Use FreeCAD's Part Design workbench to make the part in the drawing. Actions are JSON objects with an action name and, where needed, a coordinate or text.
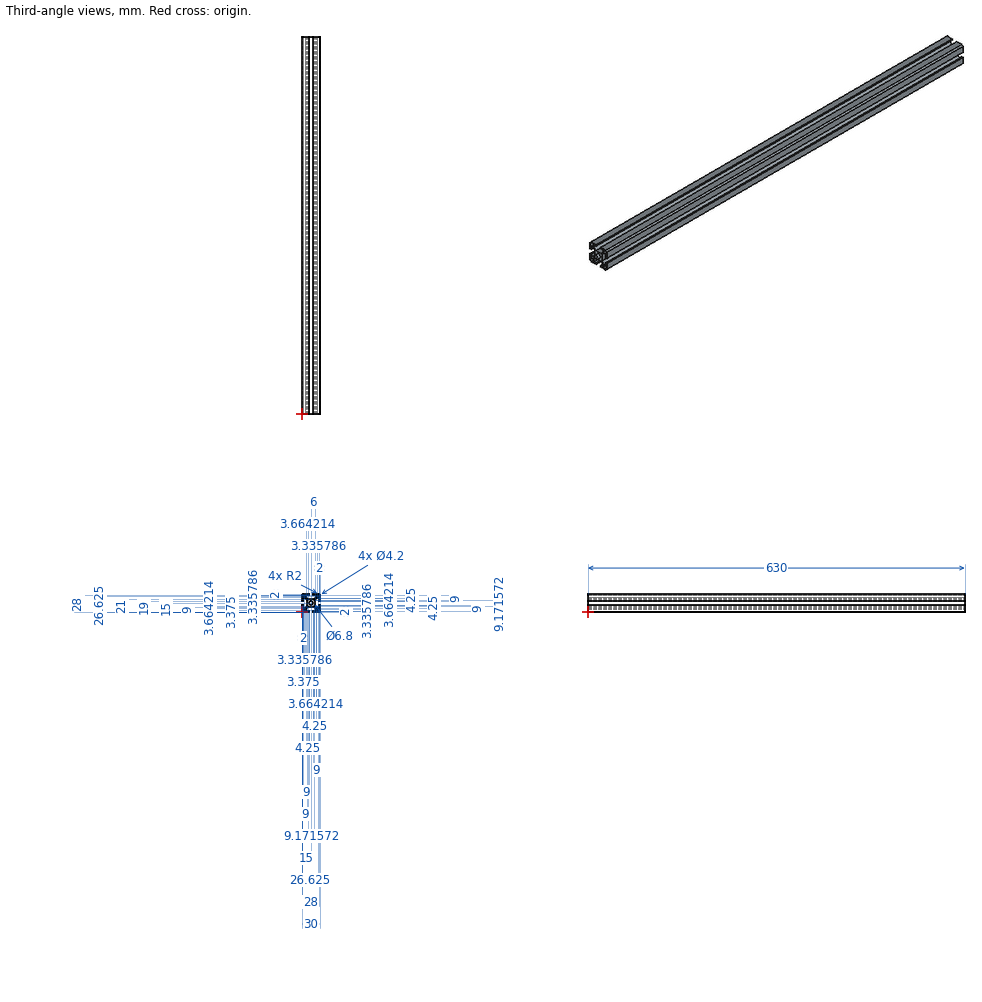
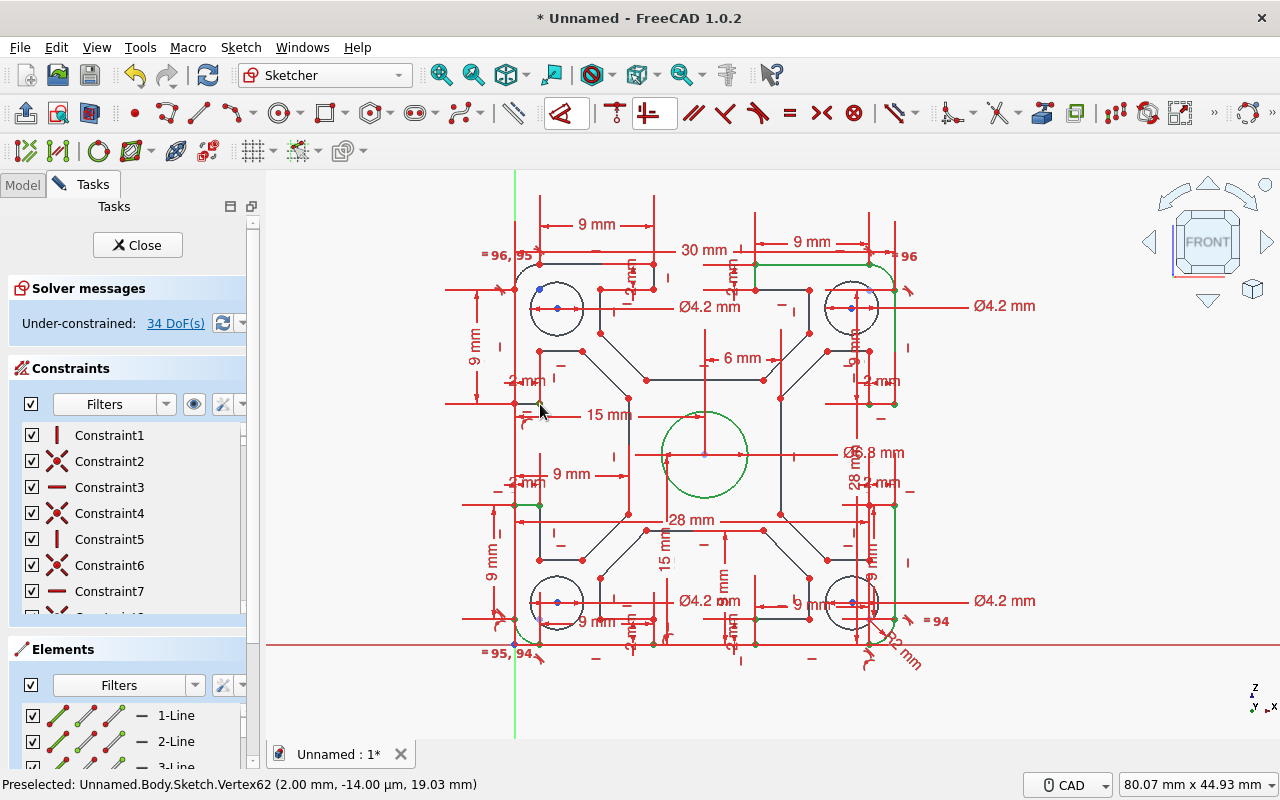
{"action": "left_click", "coordinate": [584, 114]}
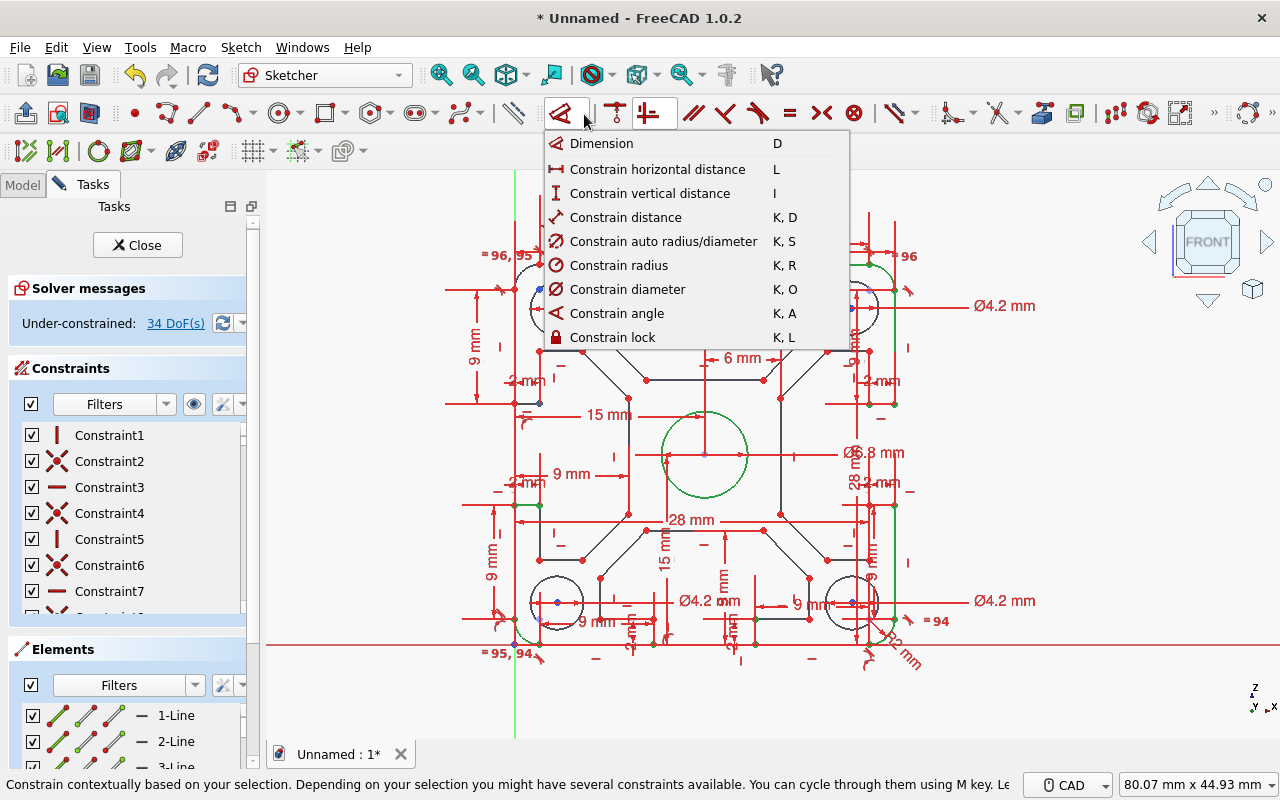
{"action": "left_click", "coordinate": [697, 193]}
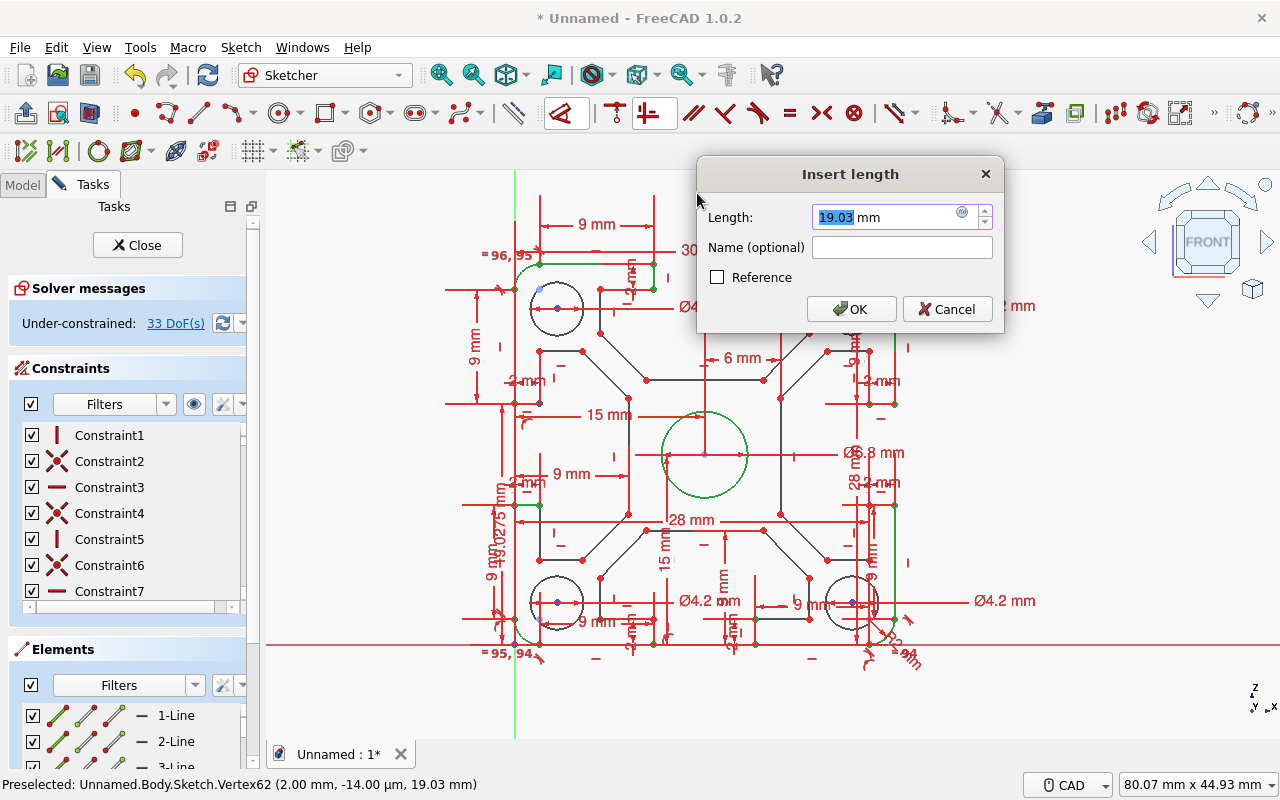
{"action": "type", "text": "19"}
{"action": "key", "text": "Return"}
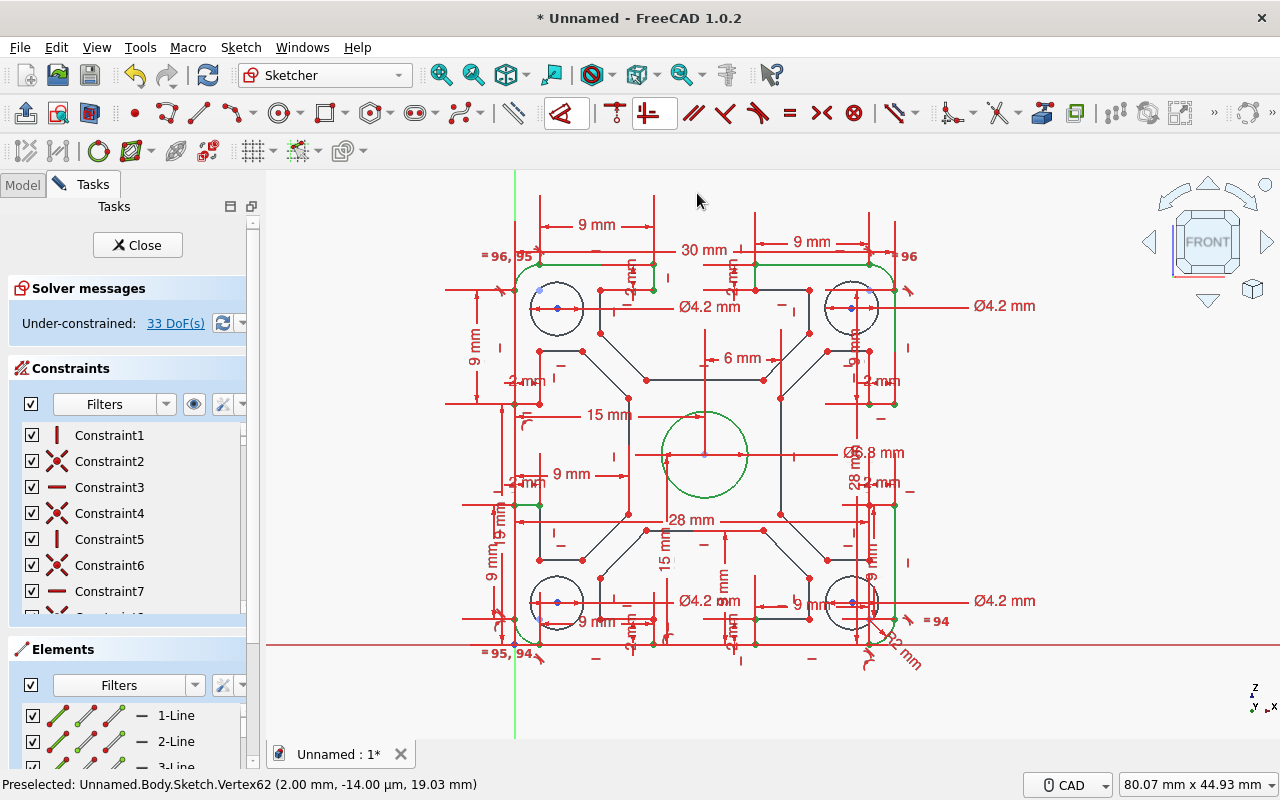
{"action": "left_click", "coordinate": [646, 380]}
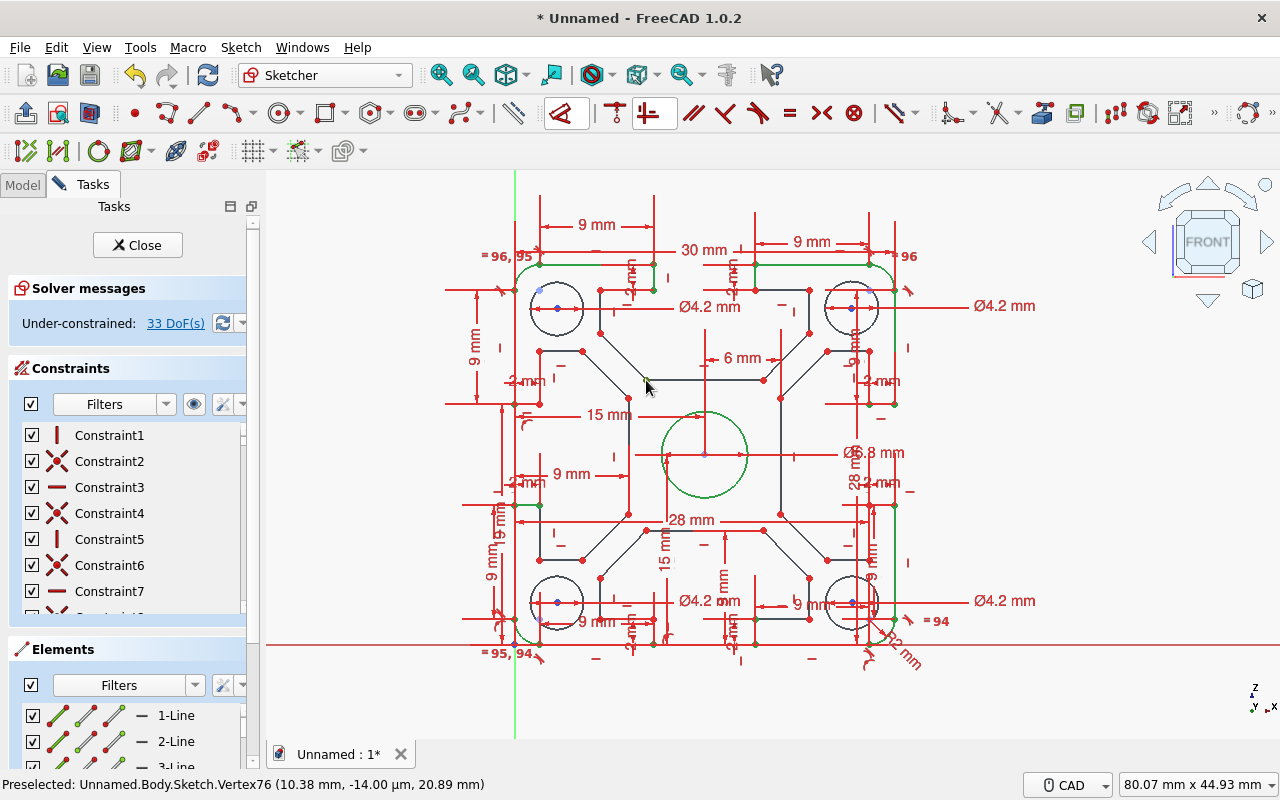
{"action": "left_click", "coordinate": [584, 114]}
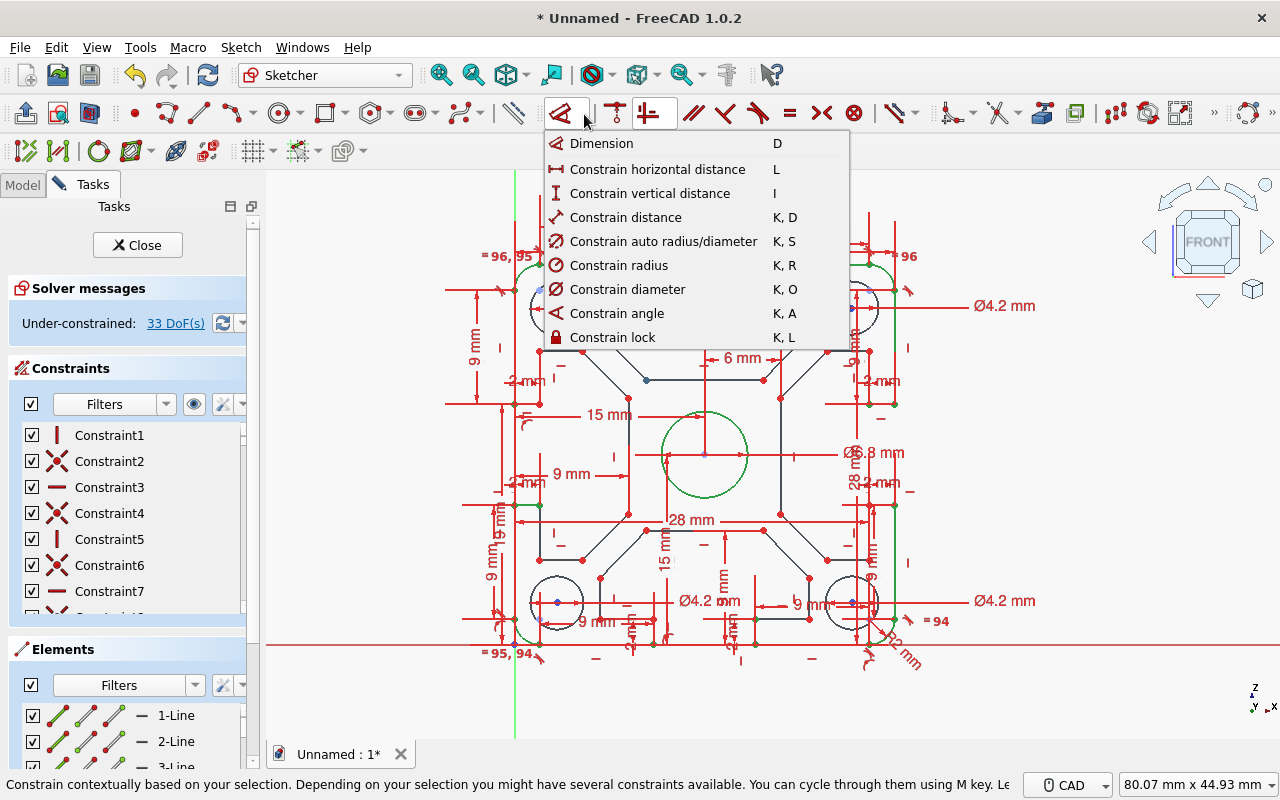
{"action": "left_click", "coordinate": [697, 193]}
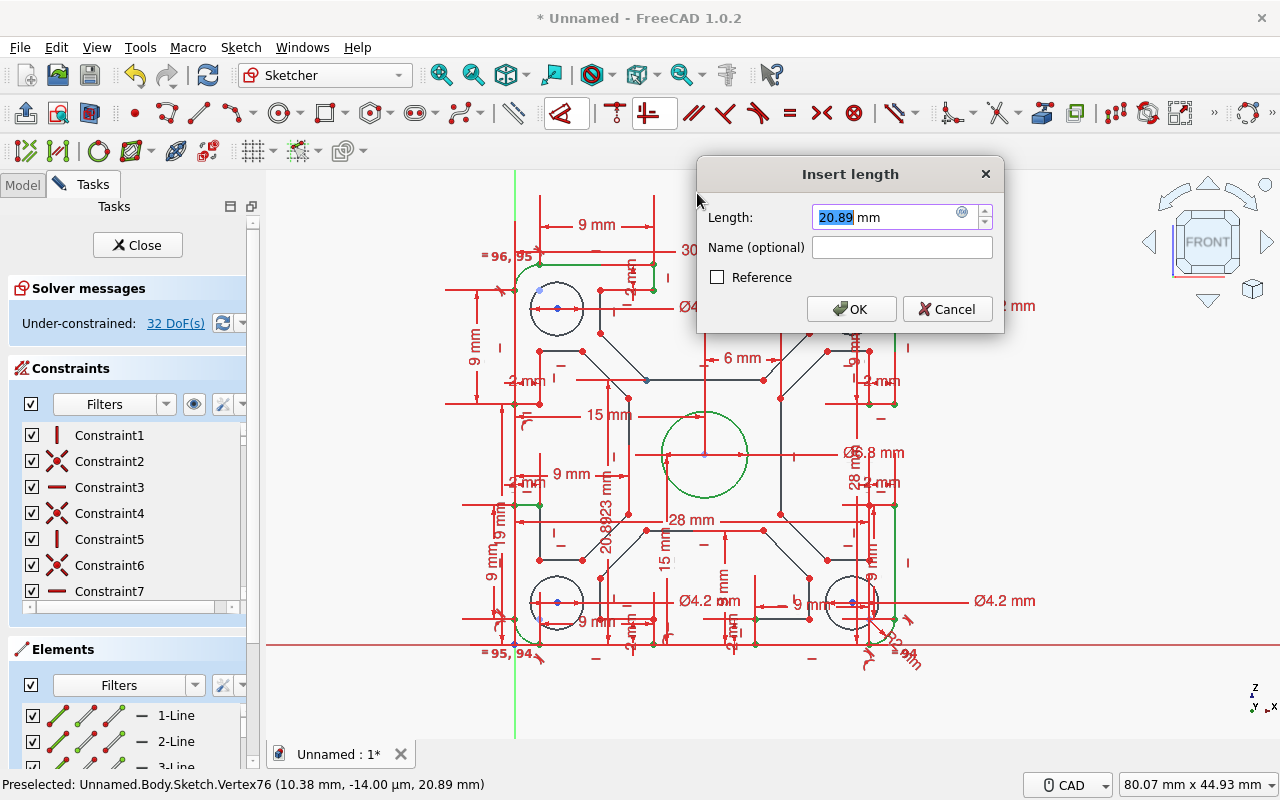
{"action": "type", "text": "21"}
{"action": "key", "text": "Return"}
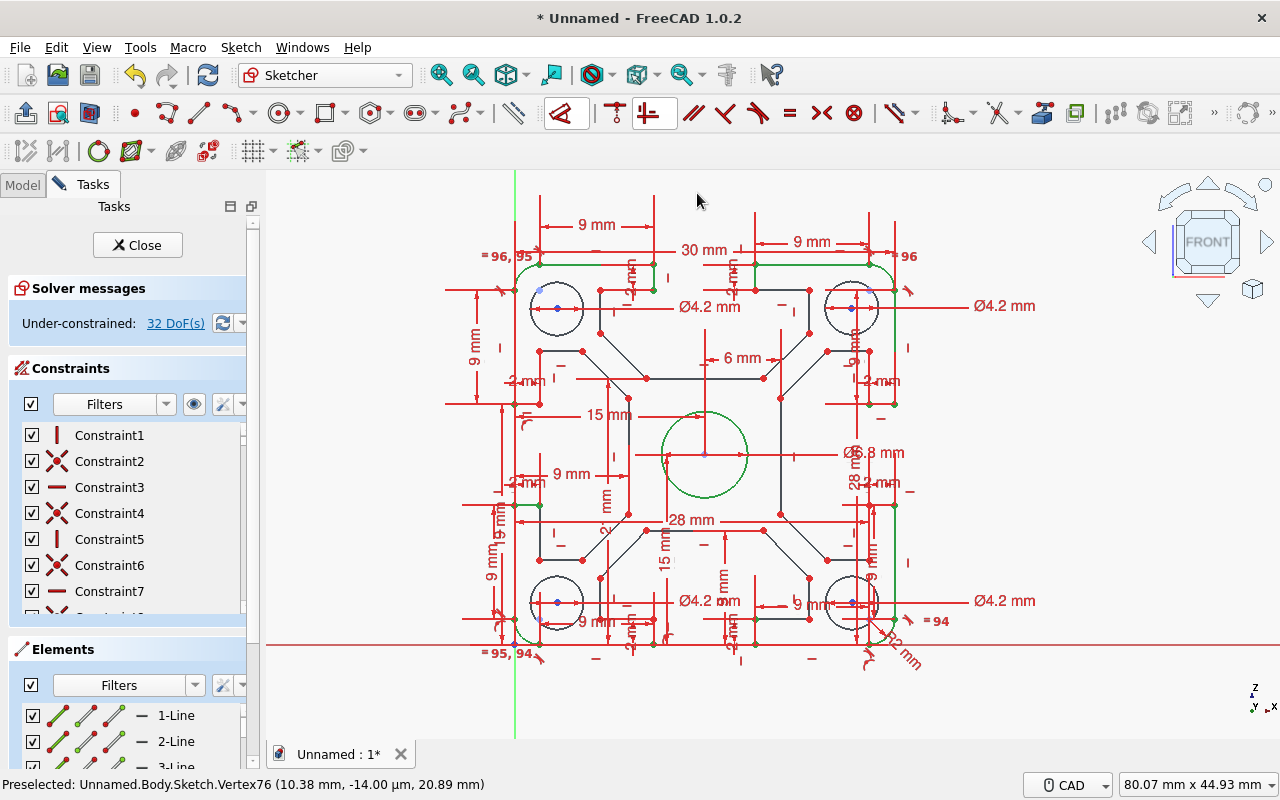
{"action": "left_click", "coordinate": [869, 367]}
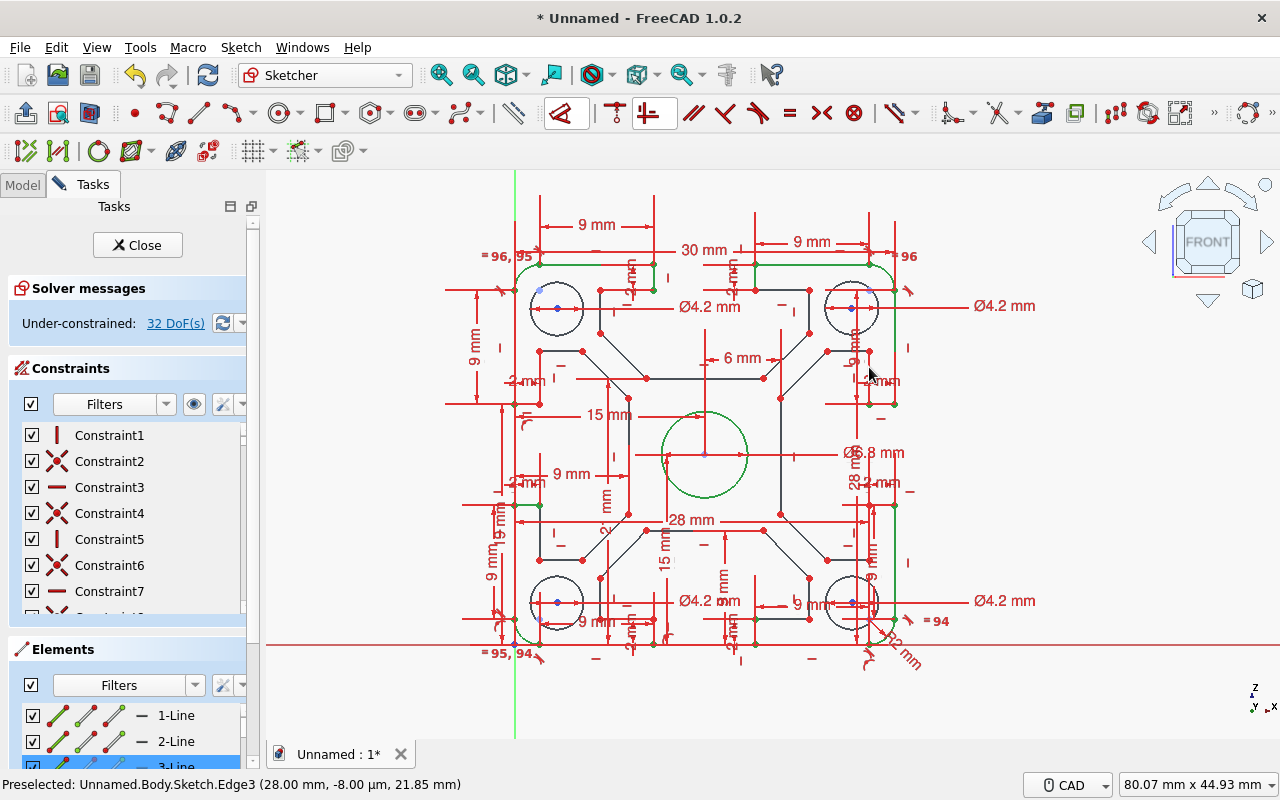
{"action": "key", "text": "i"}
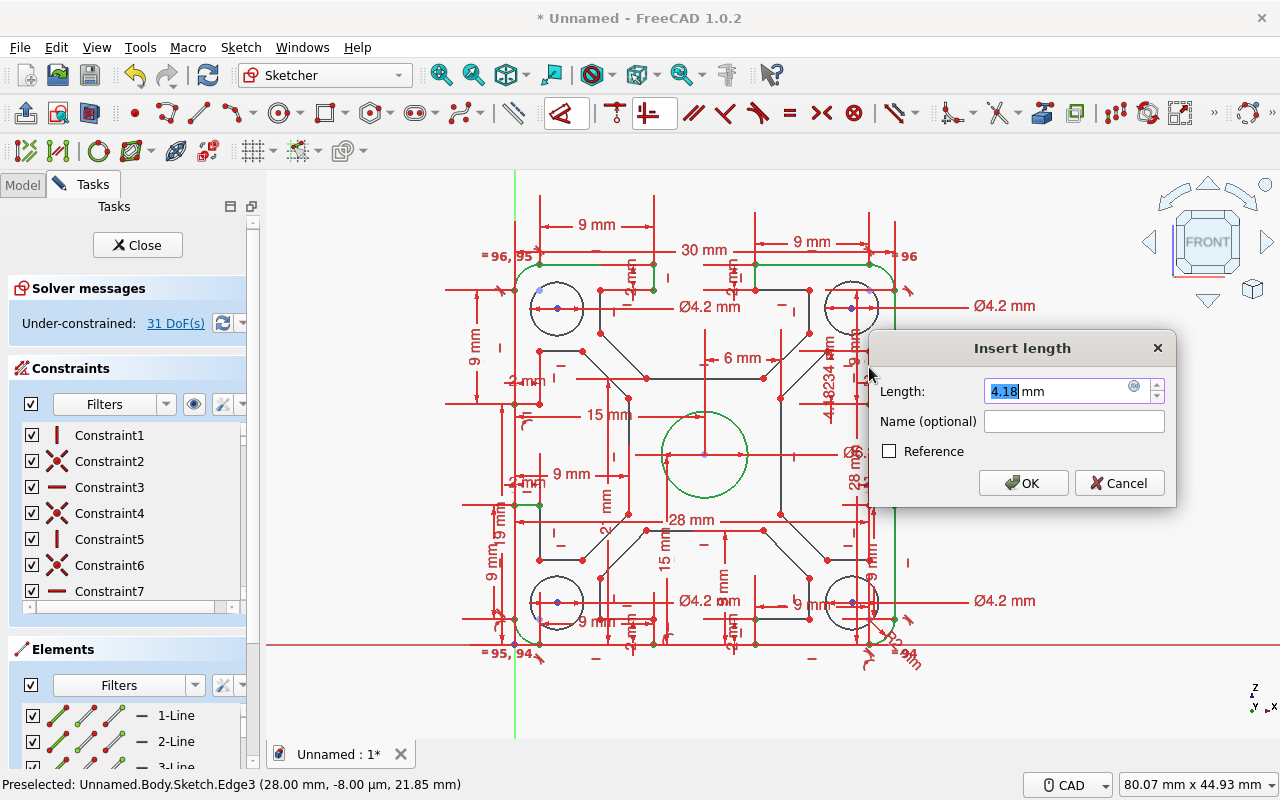
{"action": "type", "text": "4.25"}
{"action": "key", "text": "Return"}